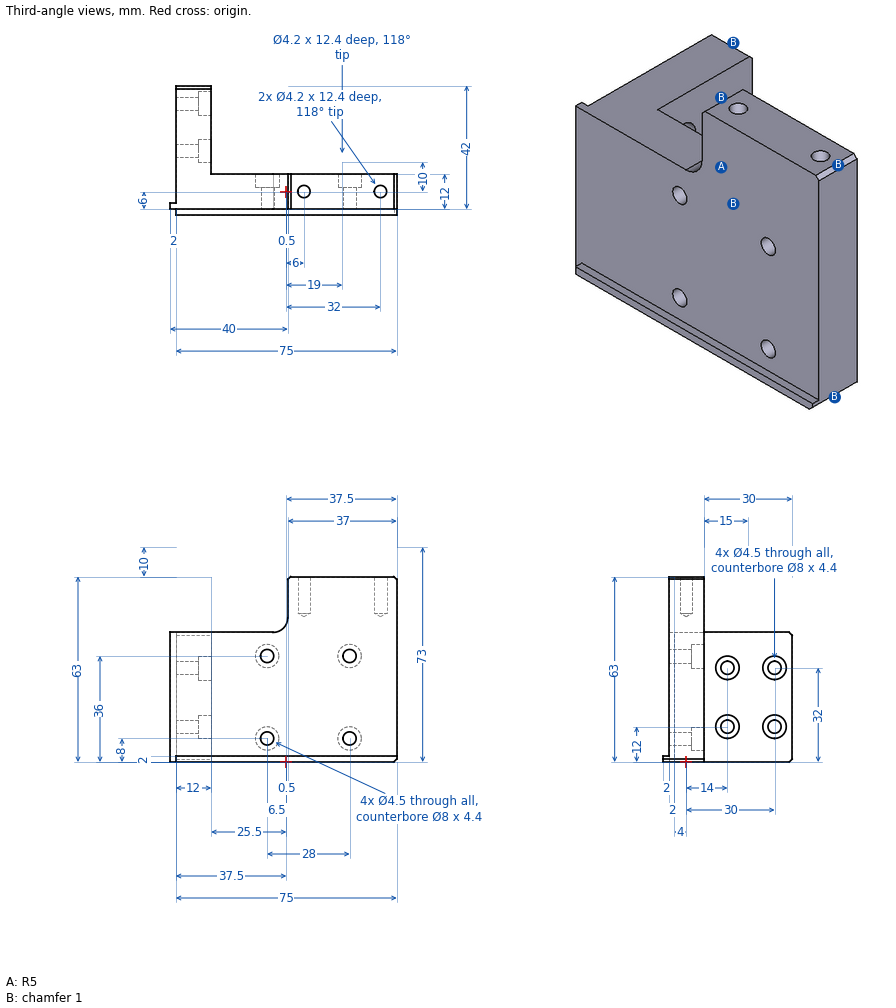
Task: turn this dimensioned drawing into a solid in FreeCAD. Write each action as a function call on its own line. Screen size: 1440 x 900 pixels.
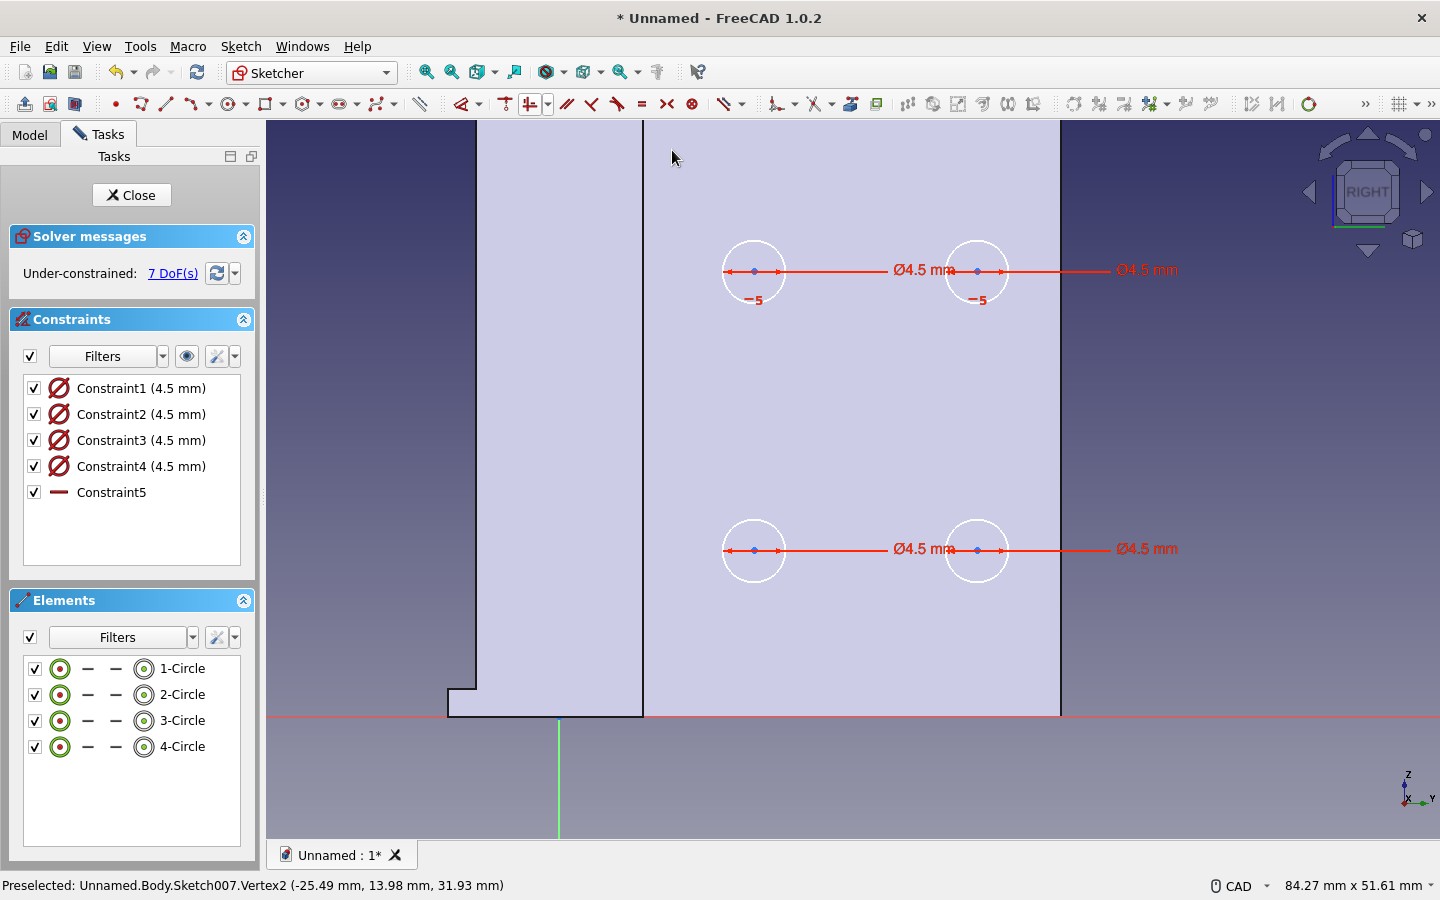
click(754, 272)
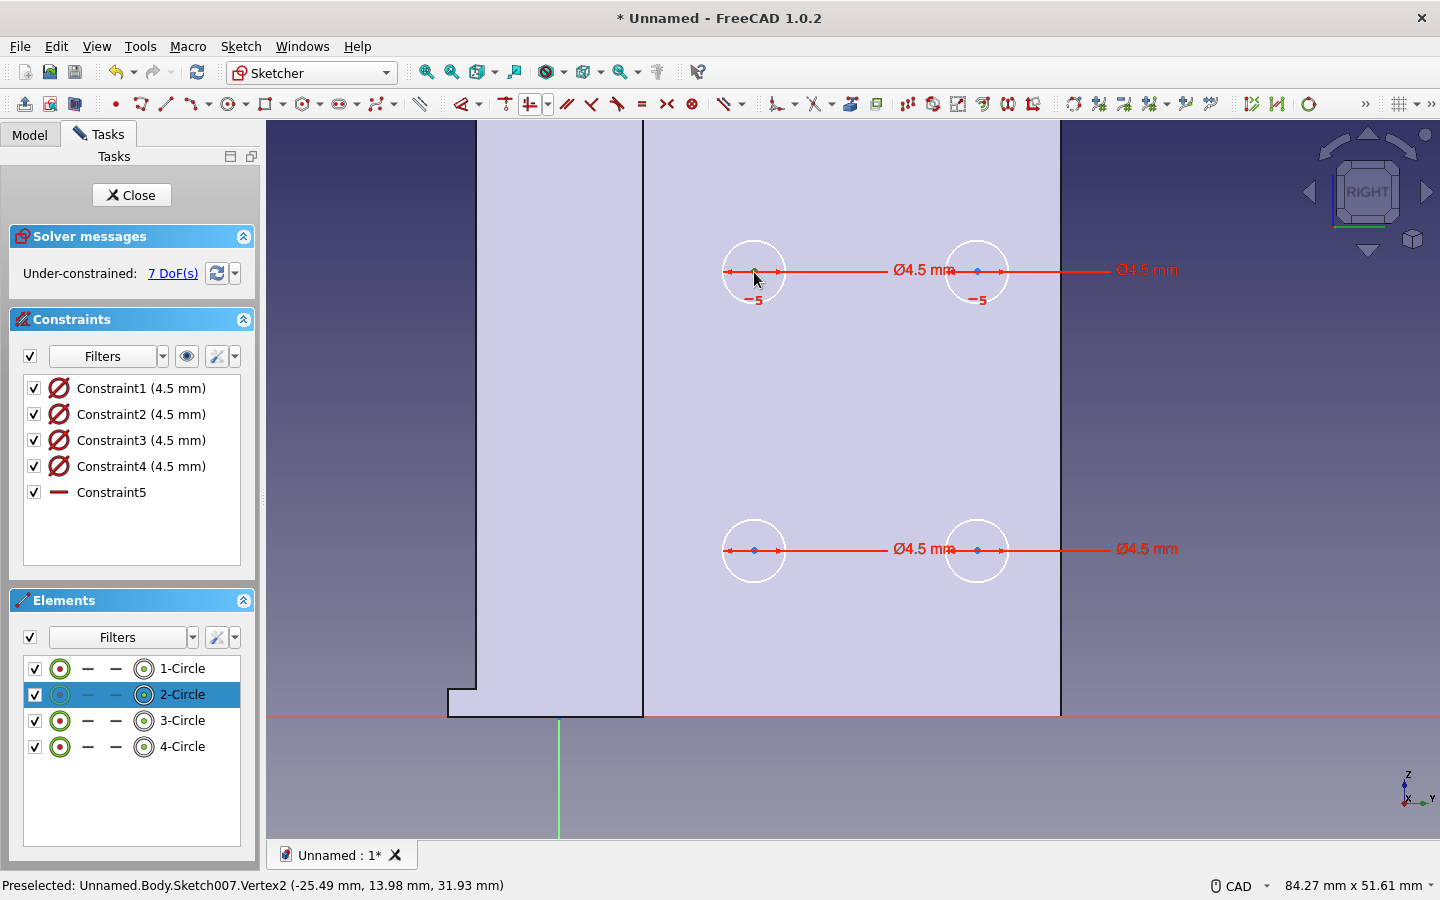
click(754, 551)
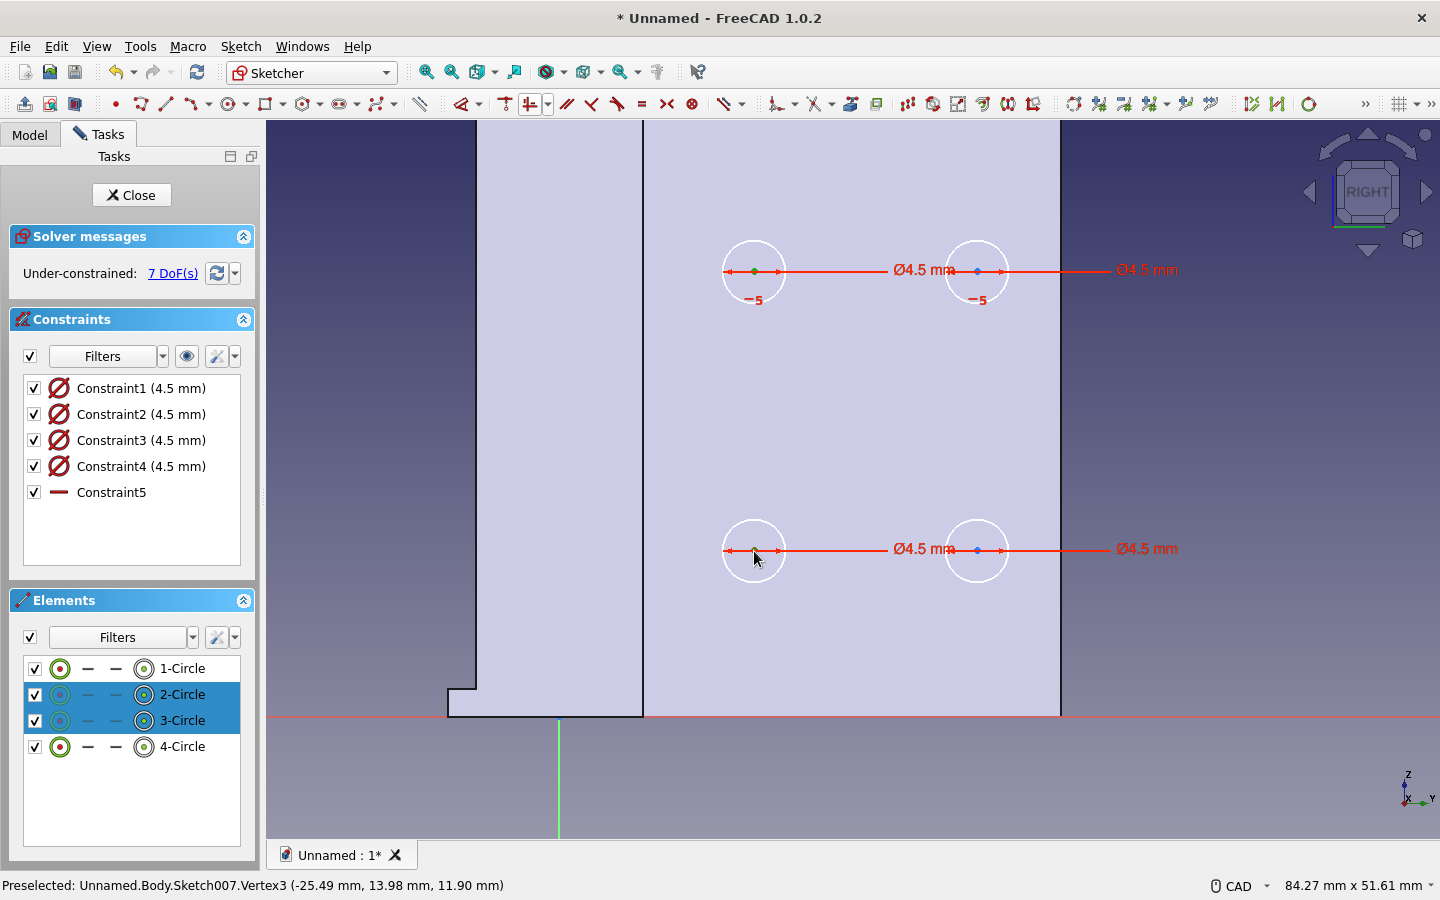
key(v)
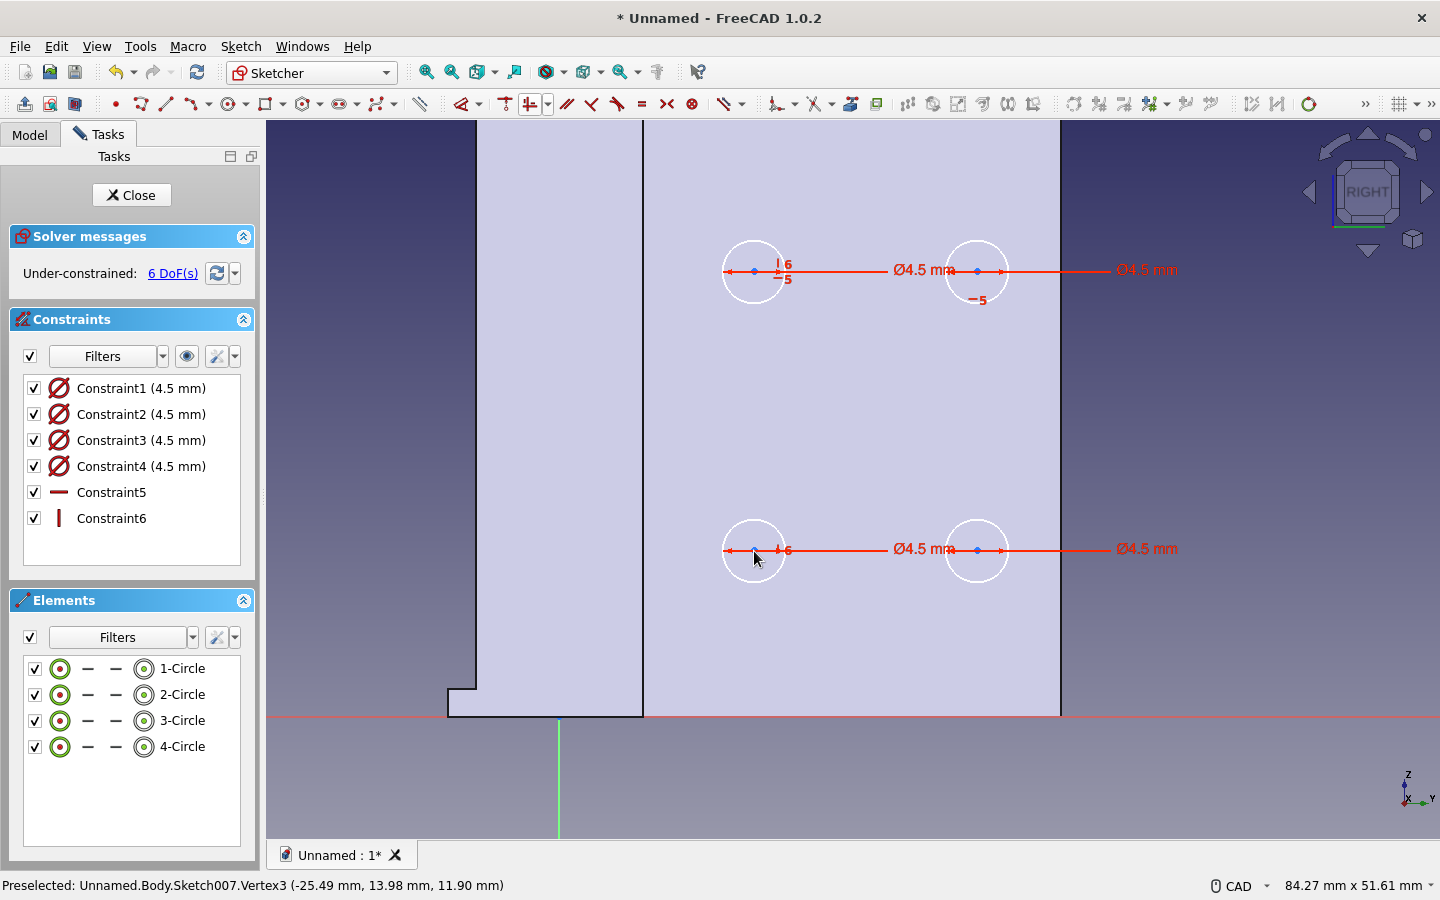
click(977, 272)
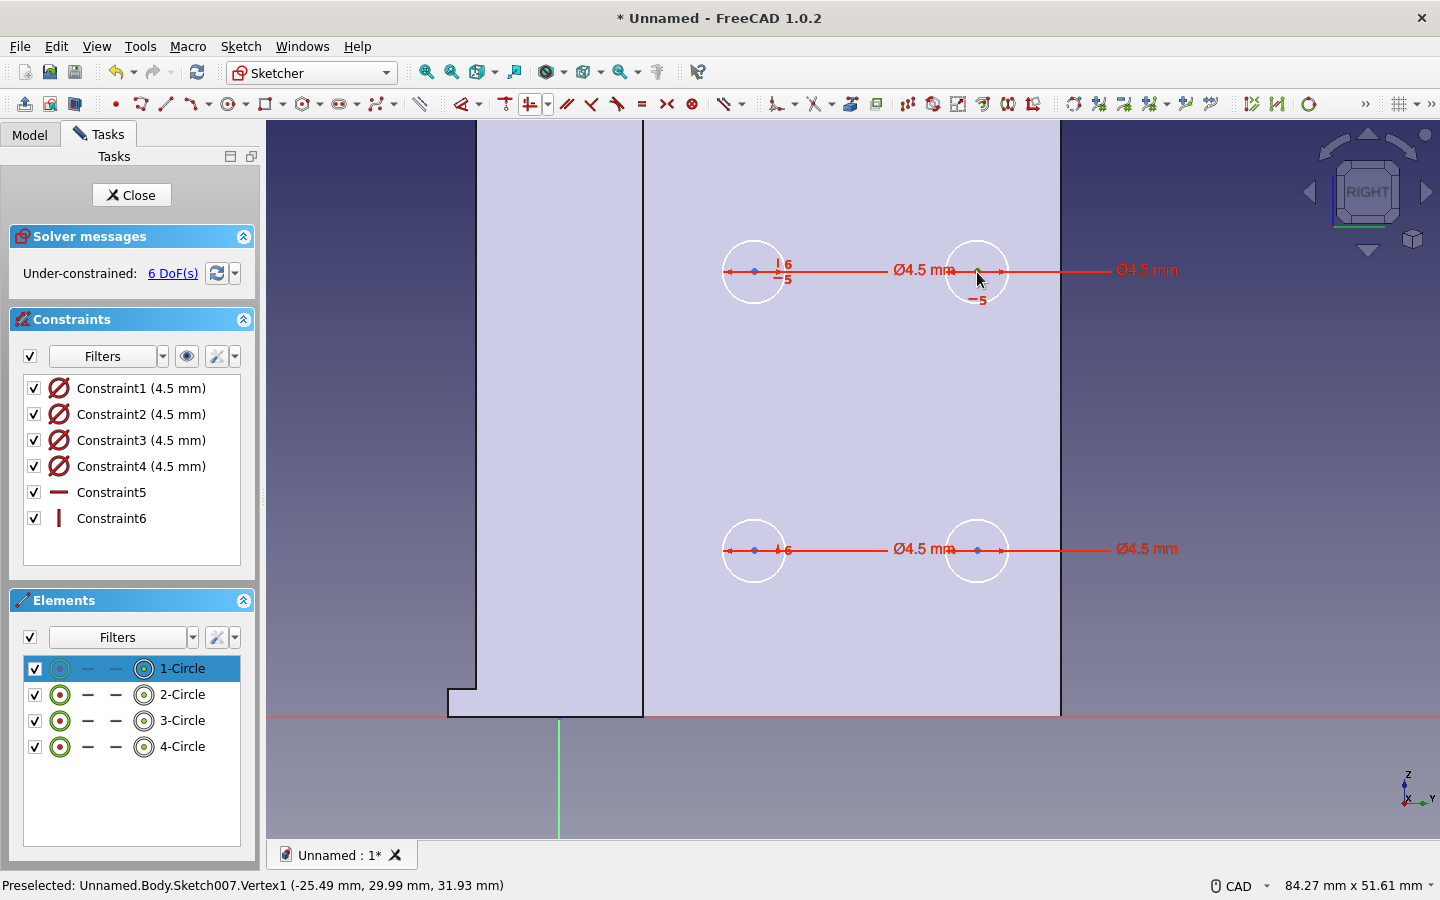
click(977, 551)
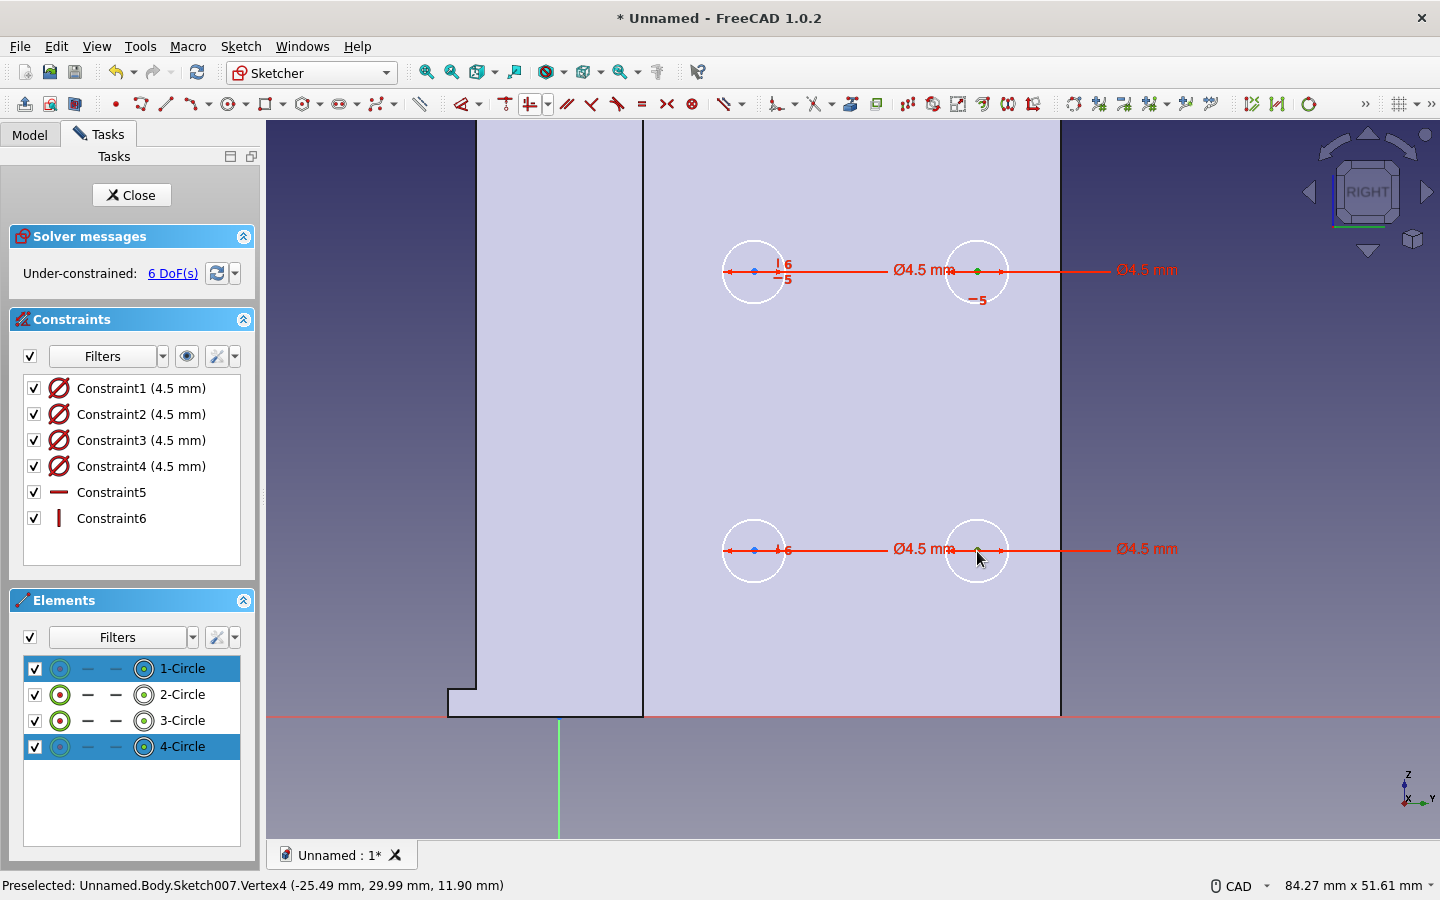
key(v)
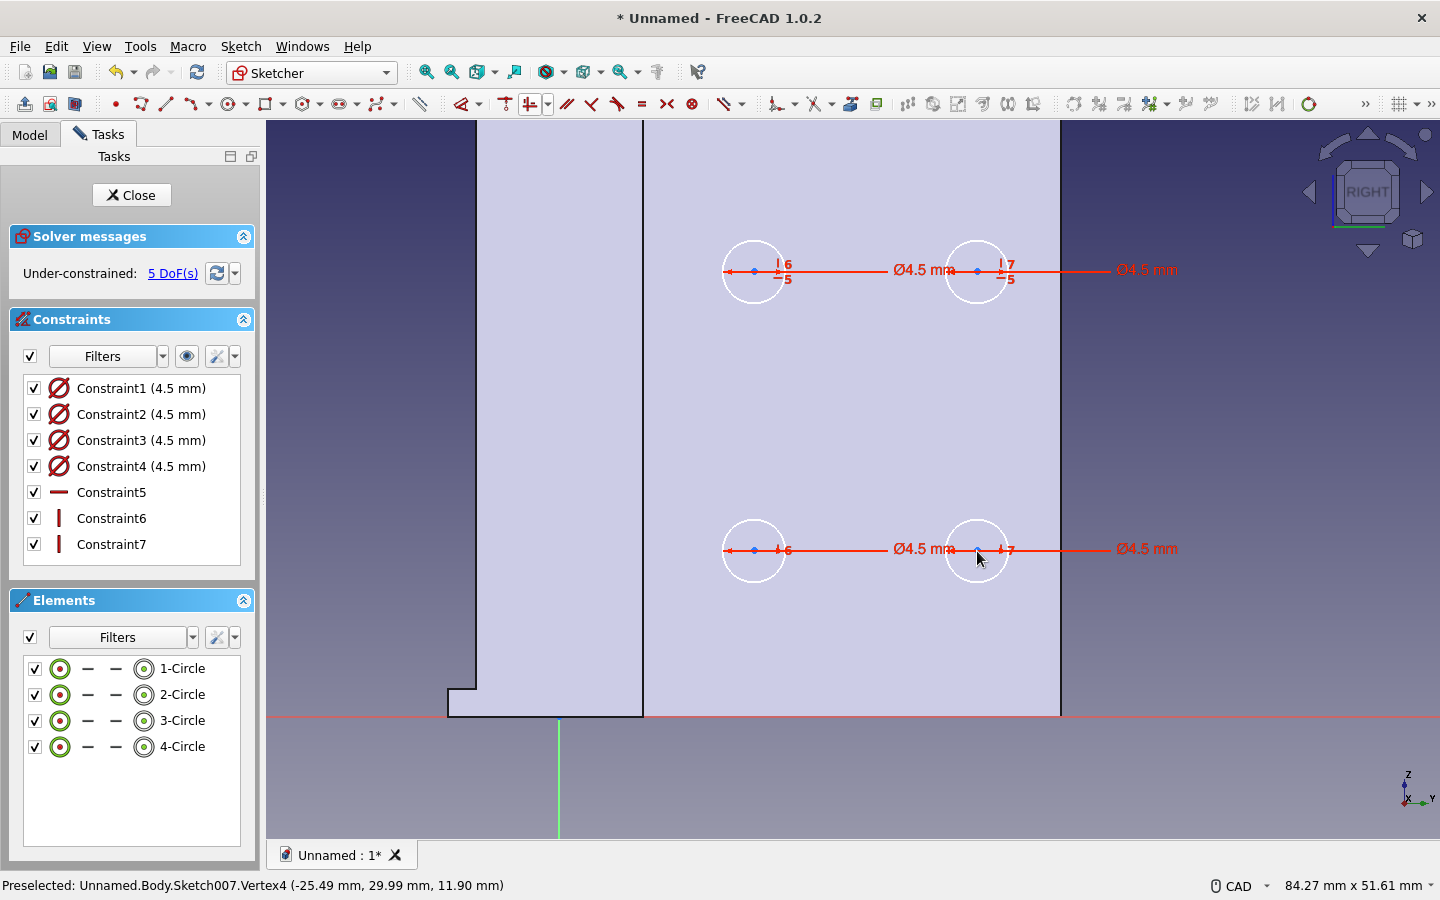
click(754, 551)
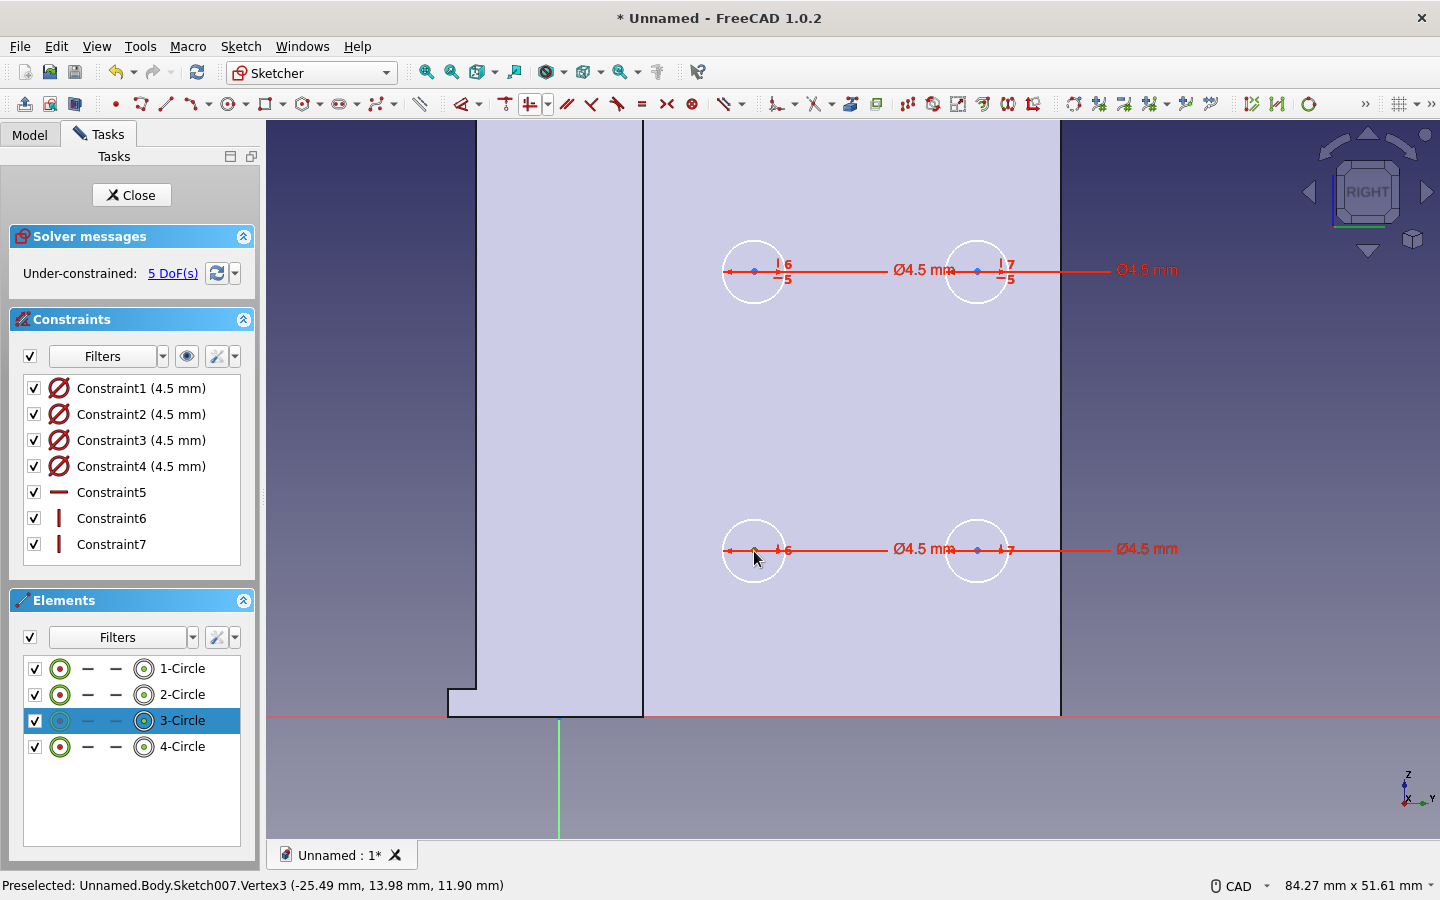
click(977, 551)